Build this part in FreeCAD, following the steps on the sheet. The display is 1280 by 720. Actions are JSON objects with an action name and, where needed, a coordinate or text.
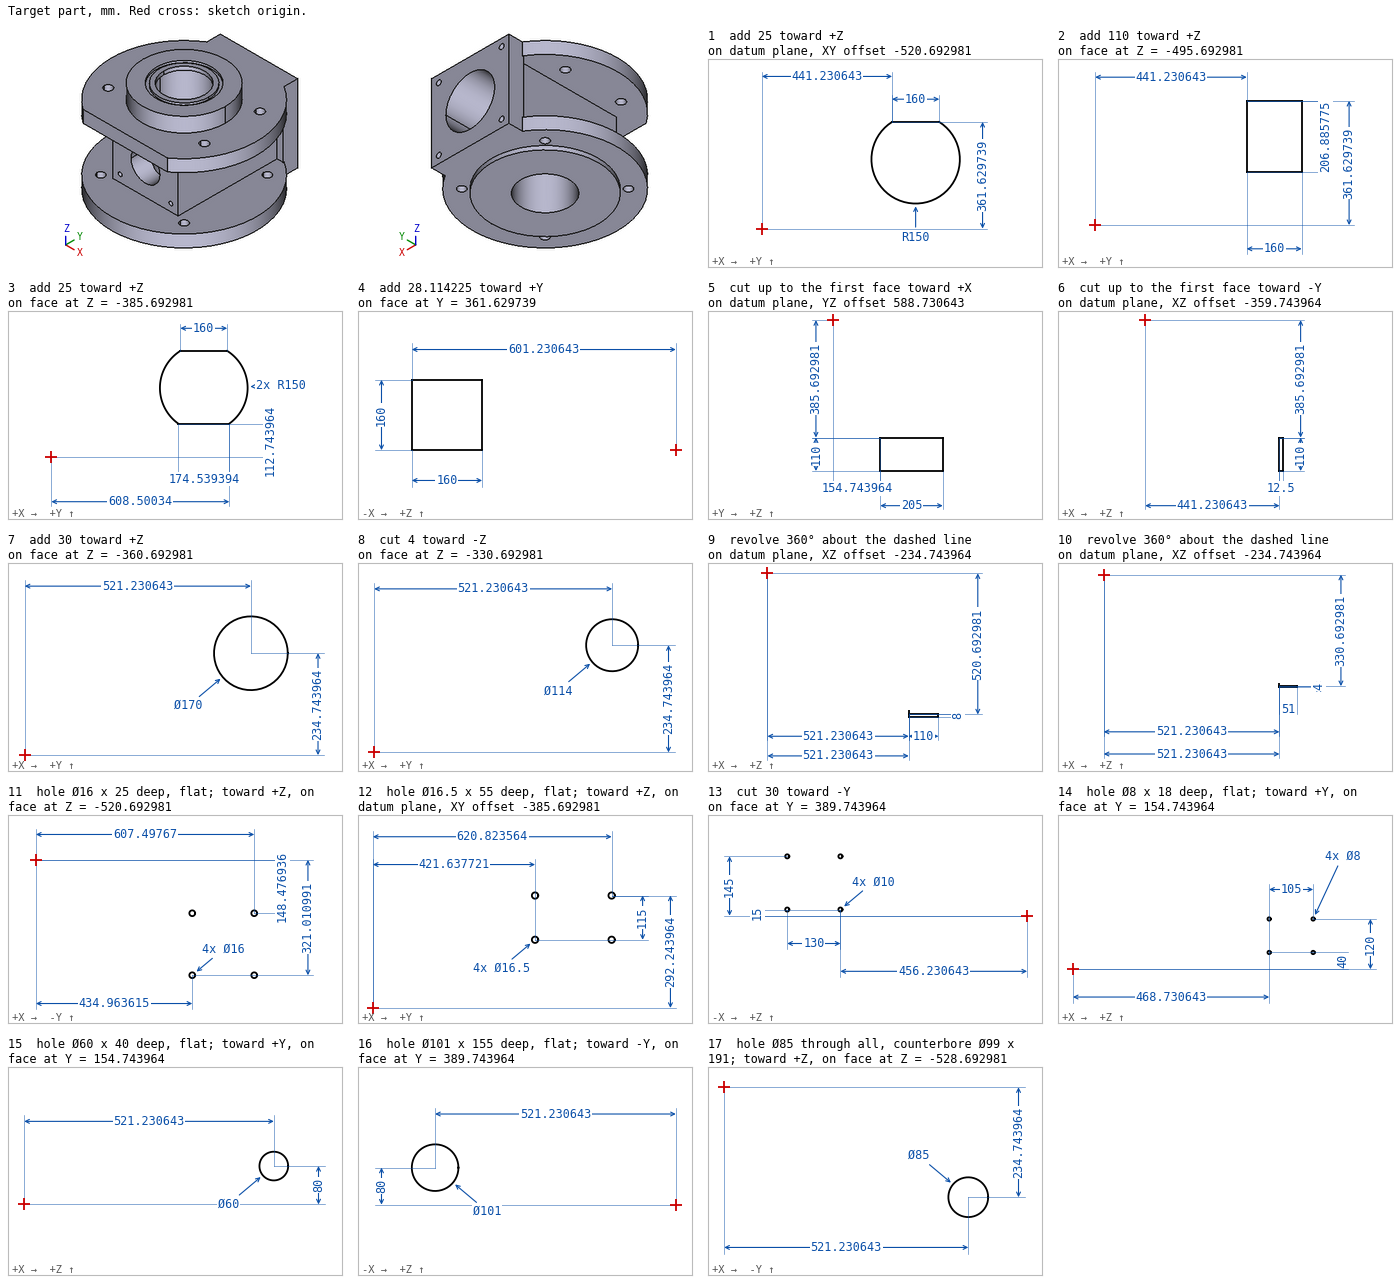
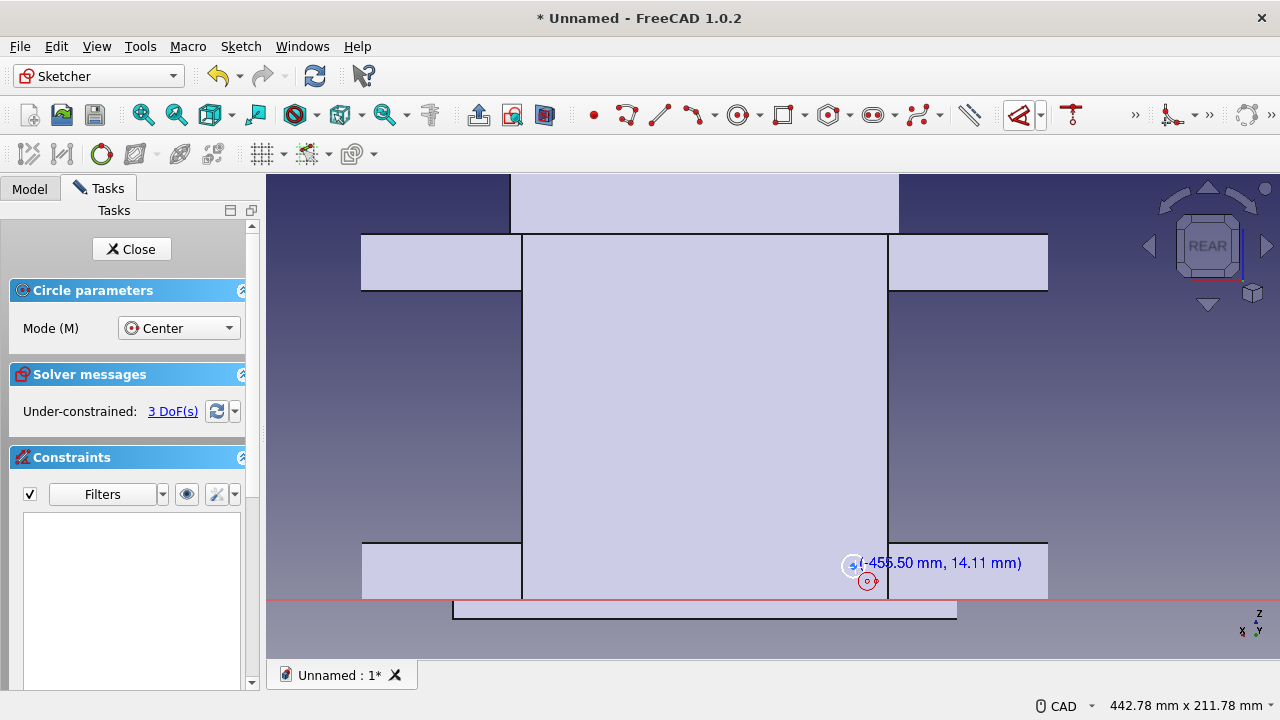
{"action": "scroll", "coordinate": [556, 566], "scroll_direction": "up", "scroll_amount": 4}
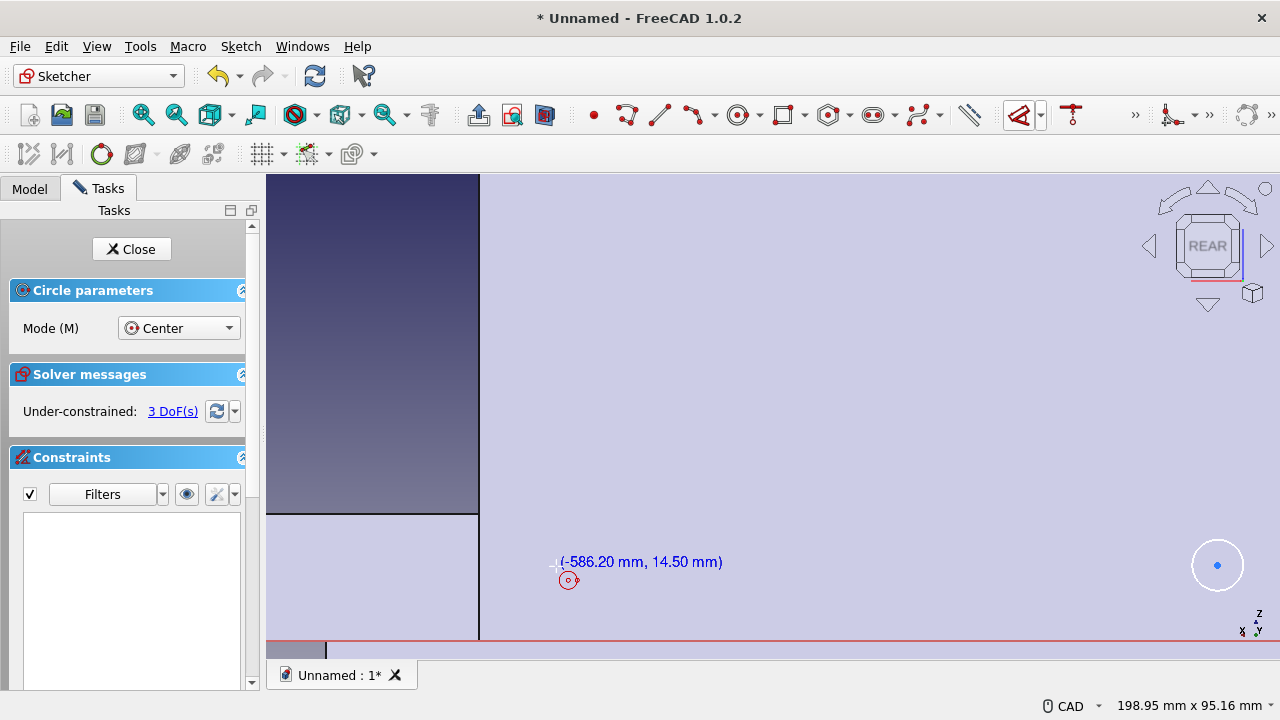
{"action": "left_click", "coordinate": [556, 565]}
{"action": "left_click", "coordinate": [574, 547]}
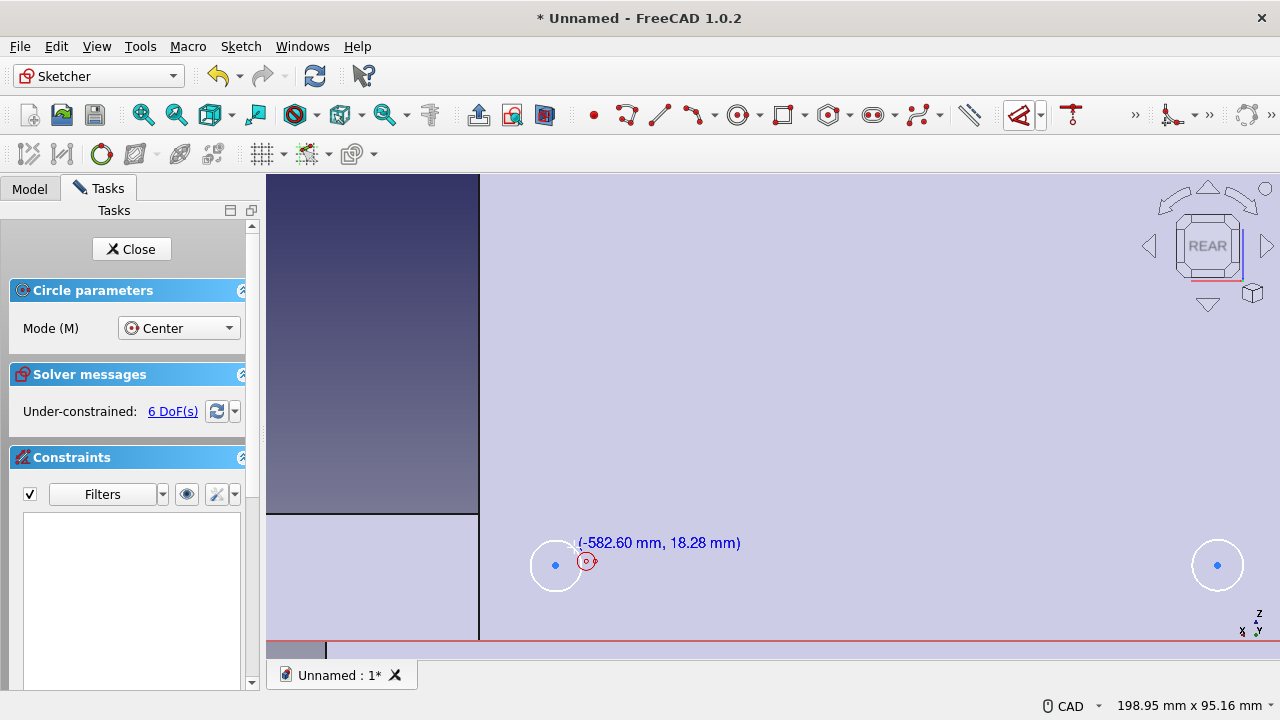
{"action": "scroll", "coordinate": [556, 566], "scroll_direction": "down", "scroll_amount": 4}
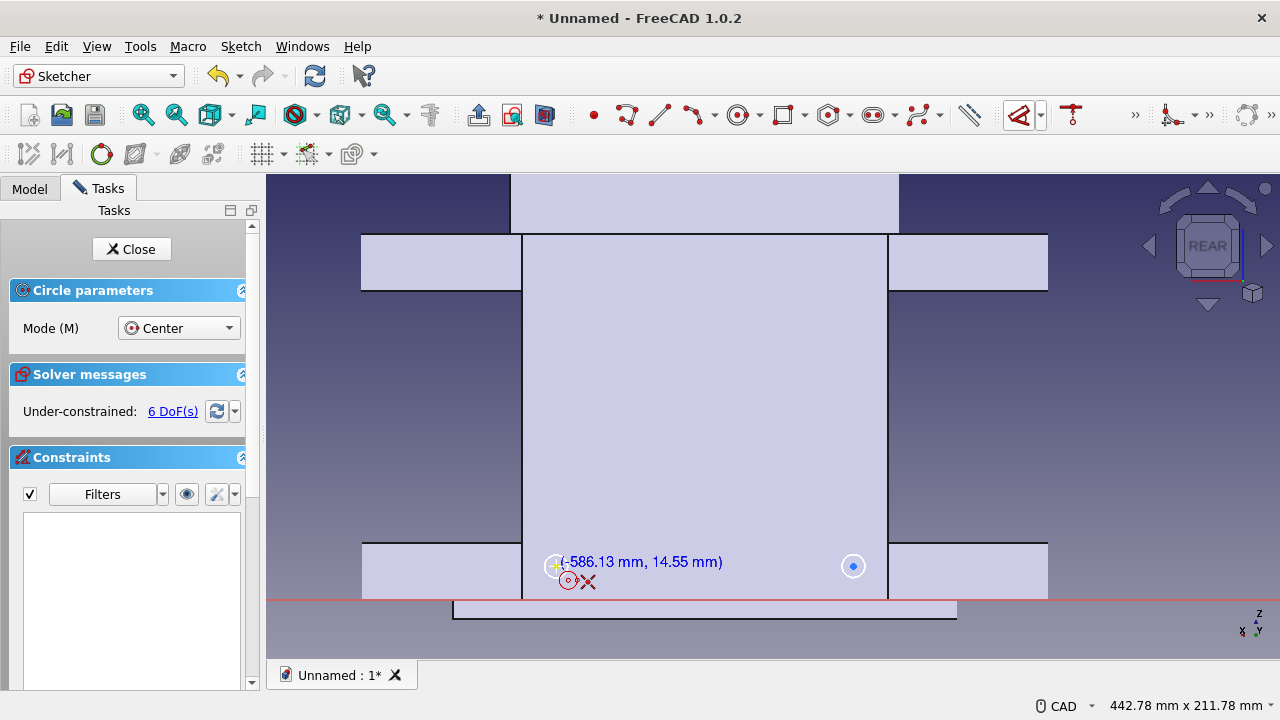
{"action": "scroll", "coordinate": [556, 268], "scroll_direction": "up", "scroll_amount": 4}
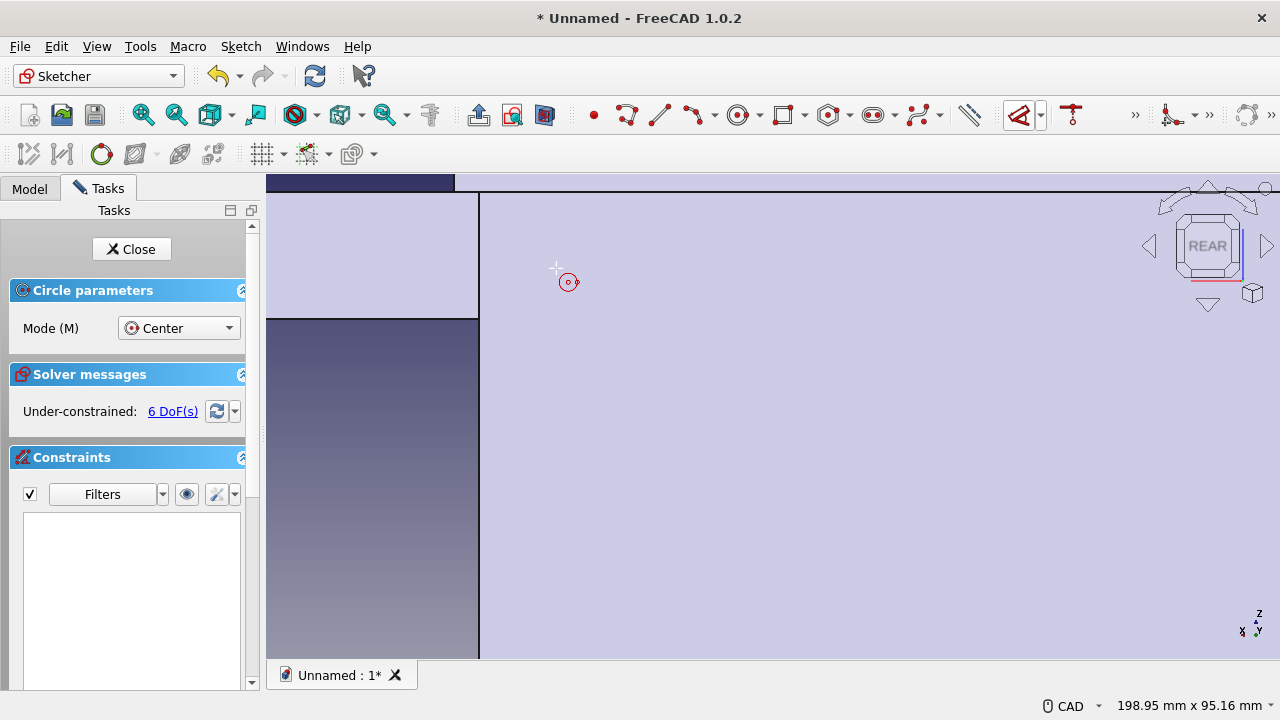
{"action": "left_click", "coordinate": [556, 268]}
{"action": "left_click", "coordinate": [574, 250]}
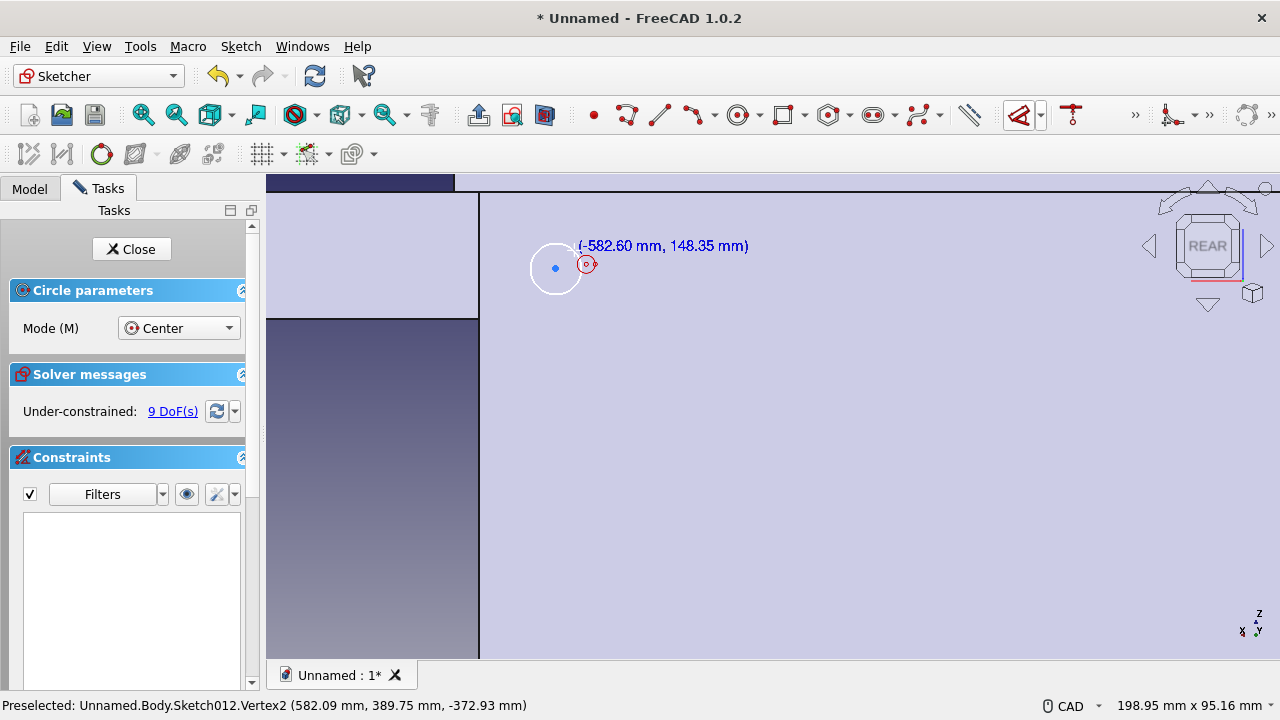
{"action": "scroll", "coordinate": [556, 267], "scroll_direction": "down", "scroll_amount": 4}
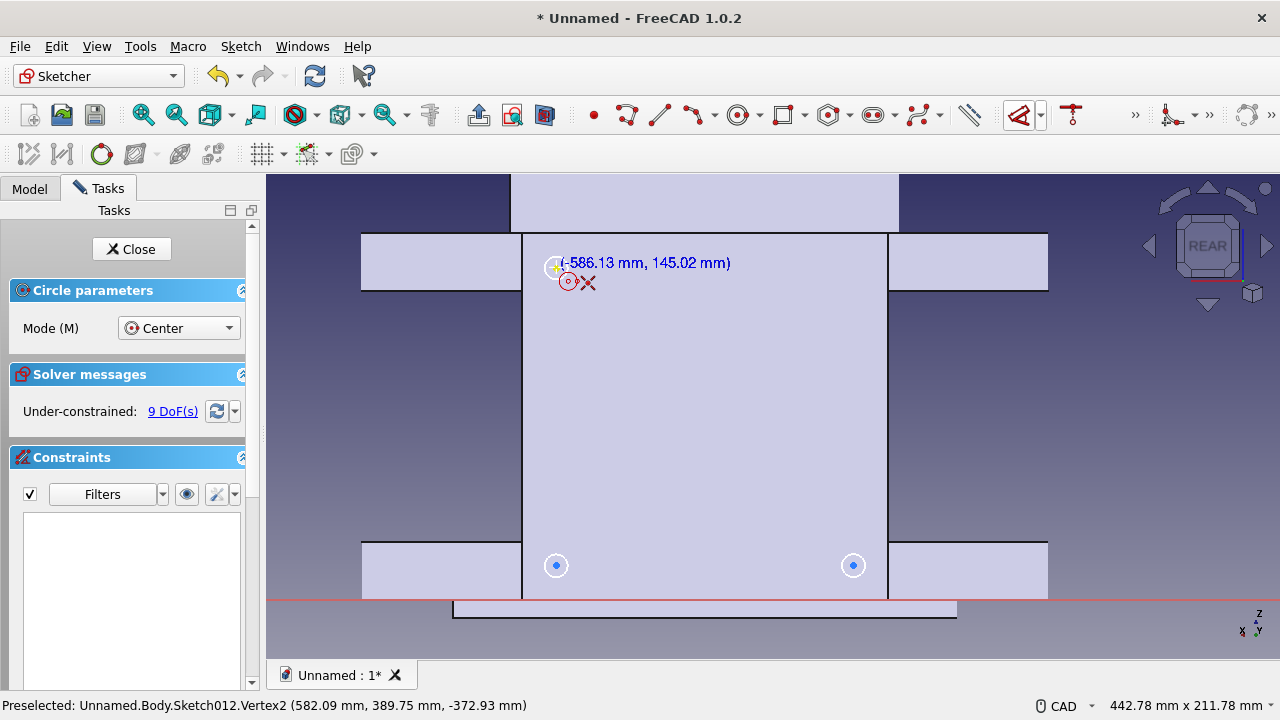
{"action": "scroll", "coordinate": [854, 268], "scroll_direction": "up", "scroll_amount": 4}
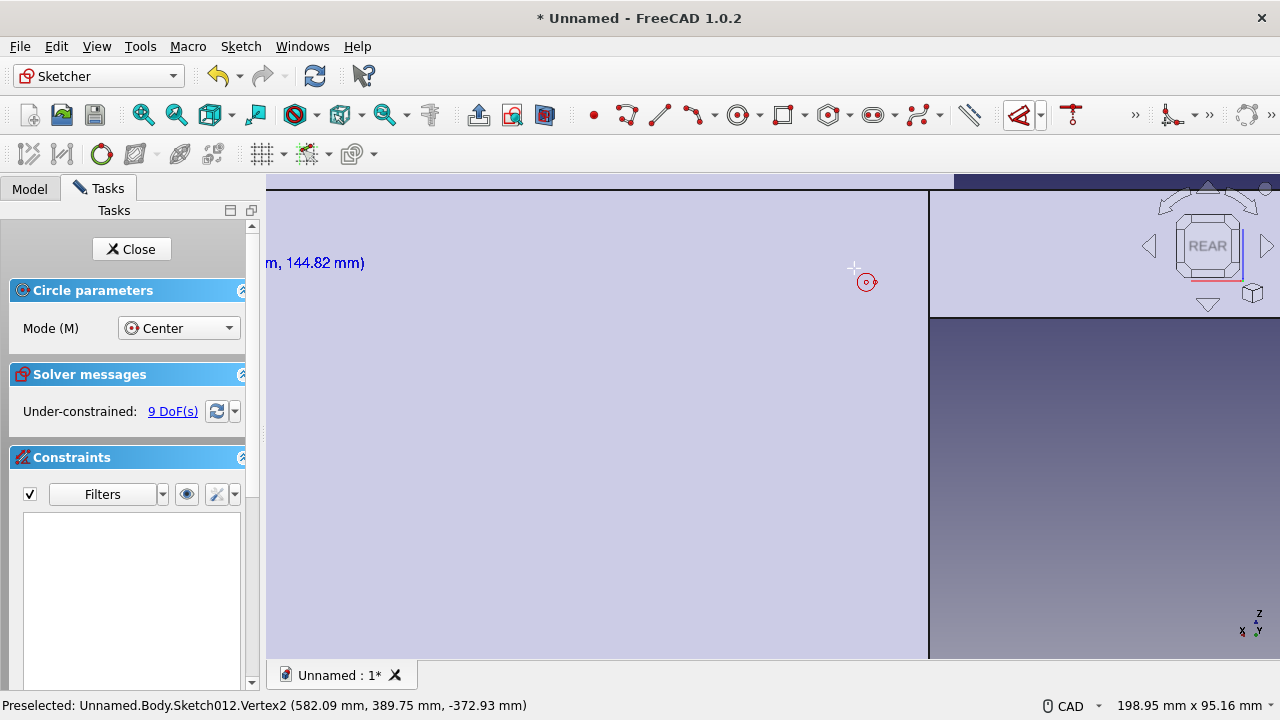
{"action": "left_click", "coordinate": [852, 267]}
{"action": "left_click", "coordinate": [871, 249]}
{"action": "key", "text": "Escape"}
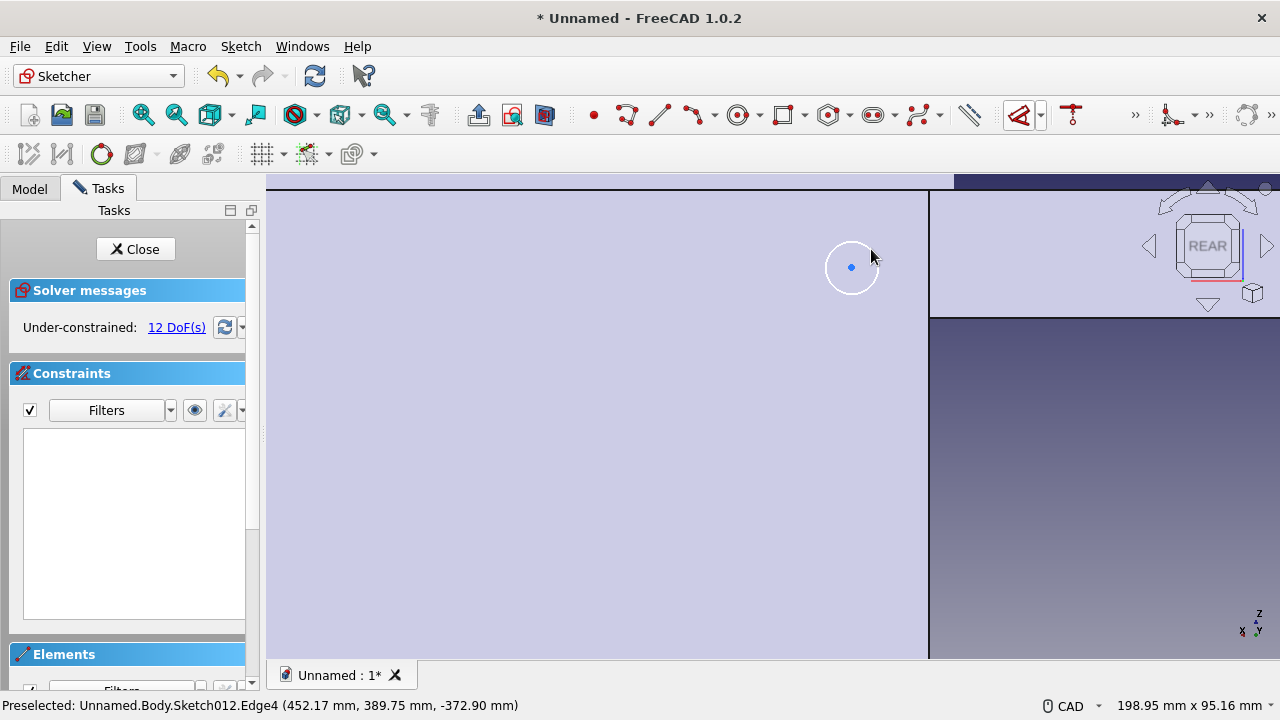
{"action": "scroll", "coordinate": [854, 268], "scroll_direction": "down", "scroll_amount": 4}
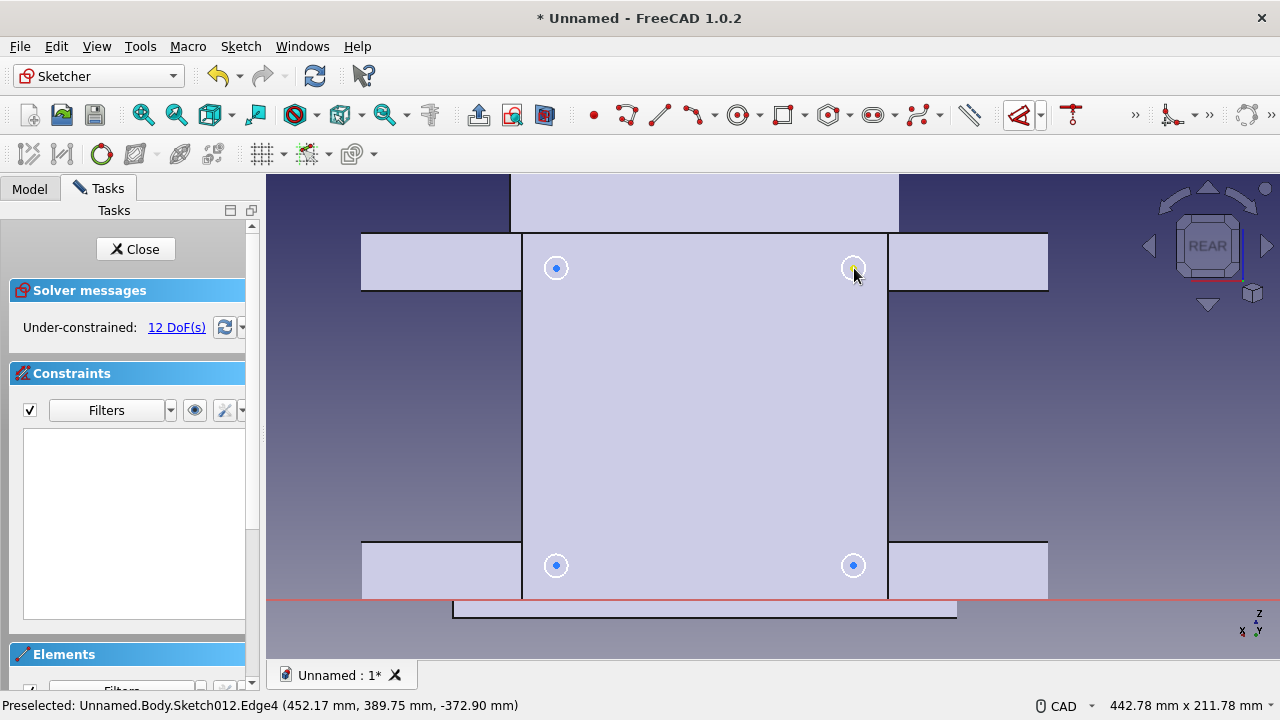
{"action": "left_click", "coordinate": [862, 557]}